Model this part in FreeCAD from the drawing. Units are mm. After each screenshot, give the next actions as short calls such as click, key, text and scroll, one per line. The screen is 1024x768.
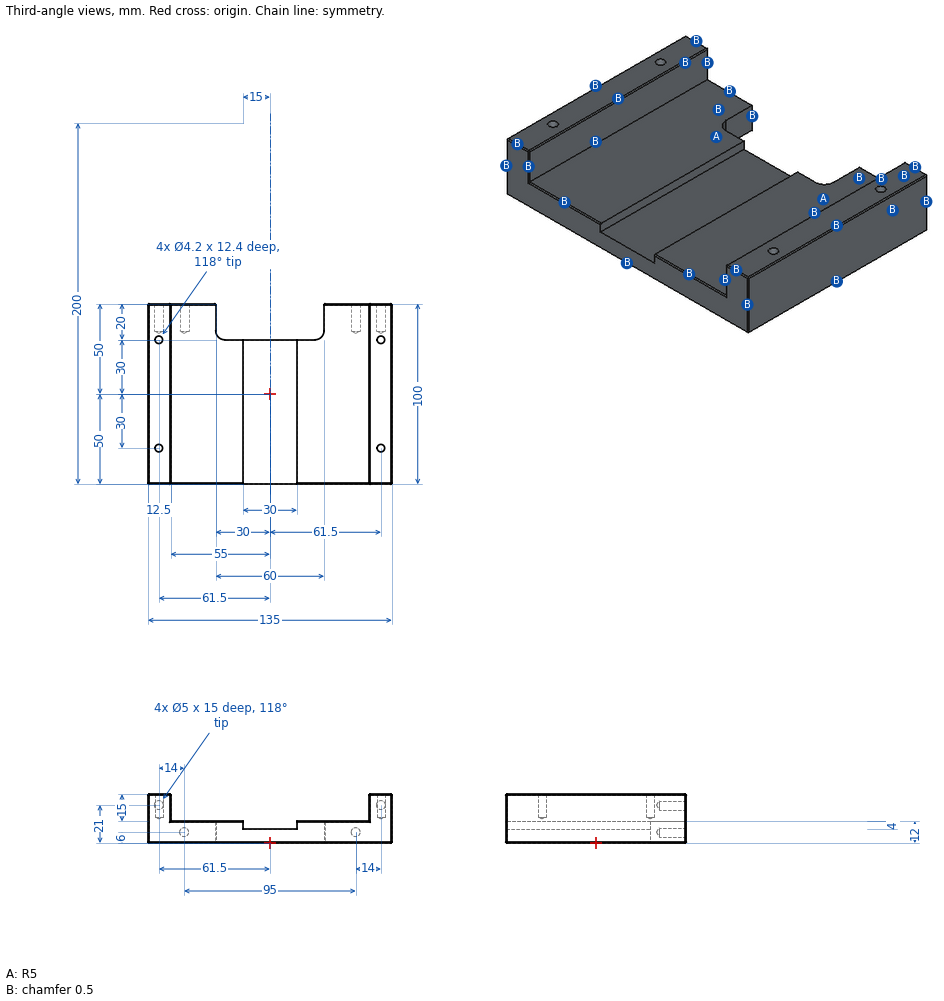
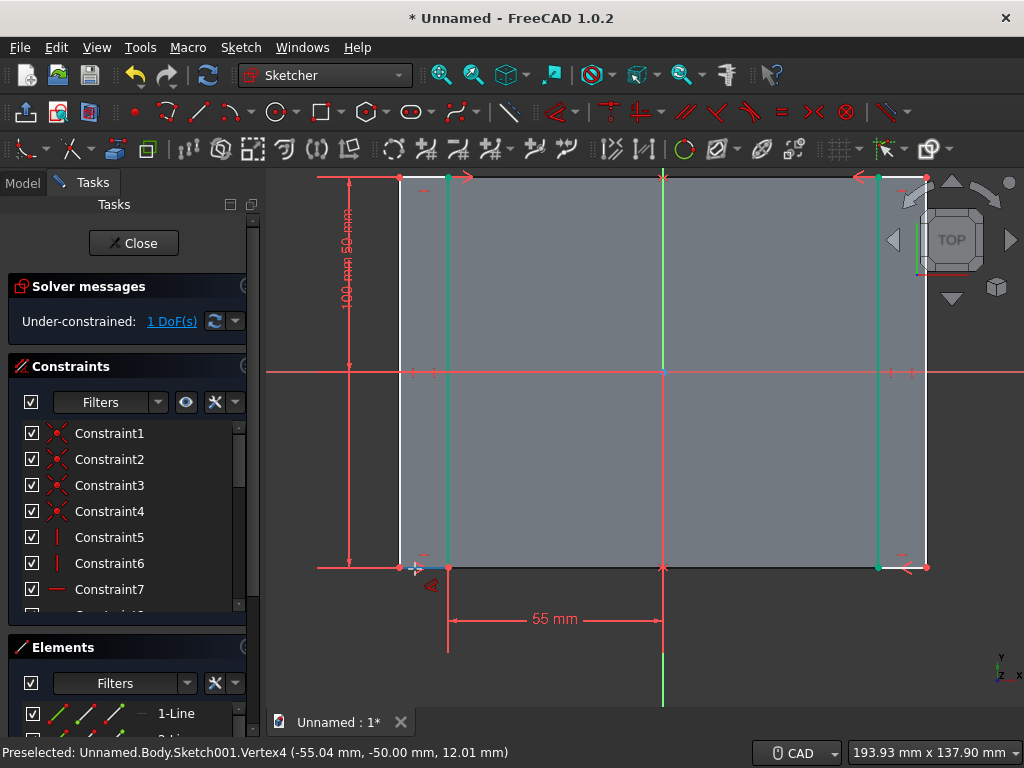
click(414, 568)
click(424, 602)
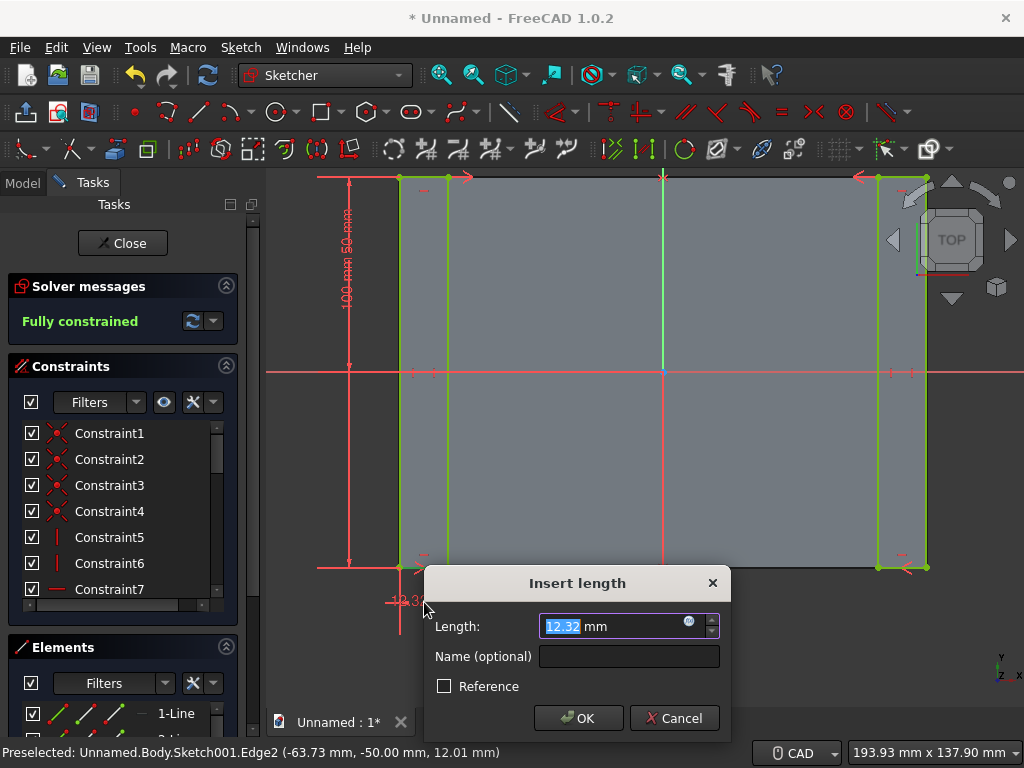
text(12.5)
key(Return)
key(Escape)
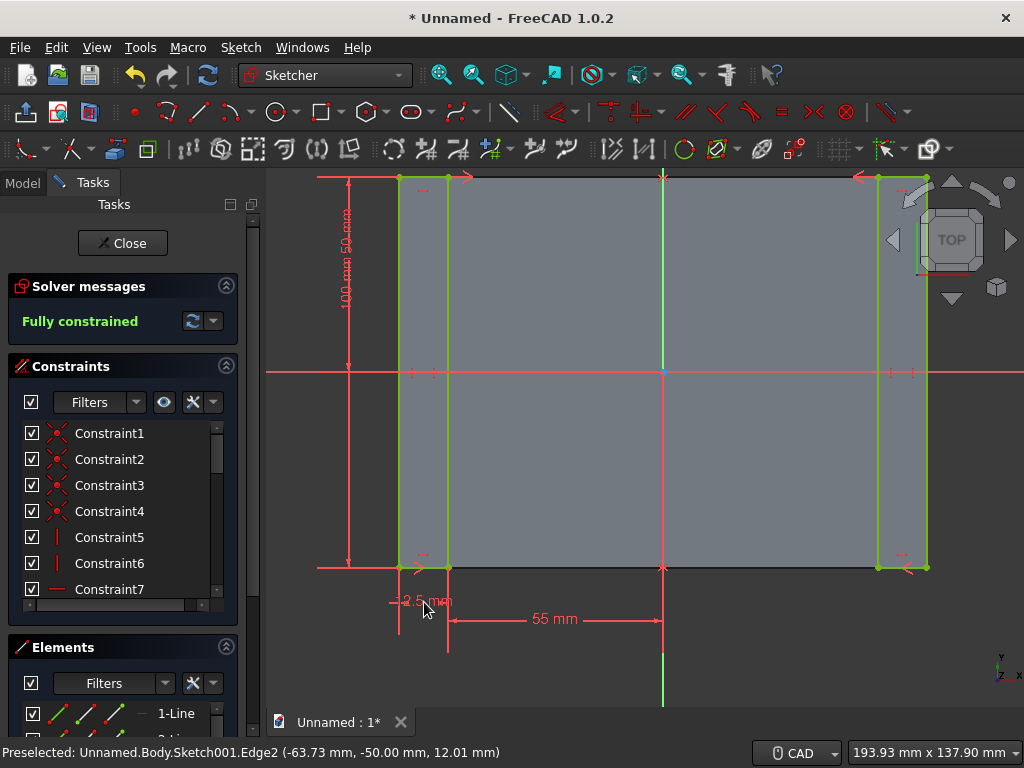
click(123, 243)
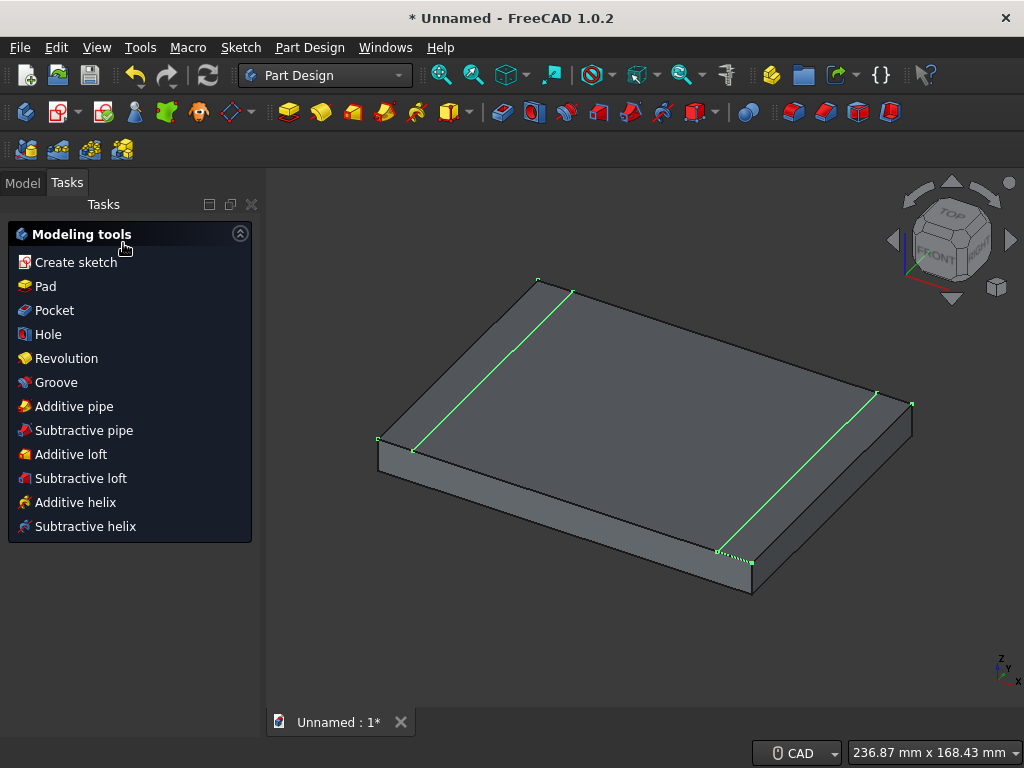
click(290, 112)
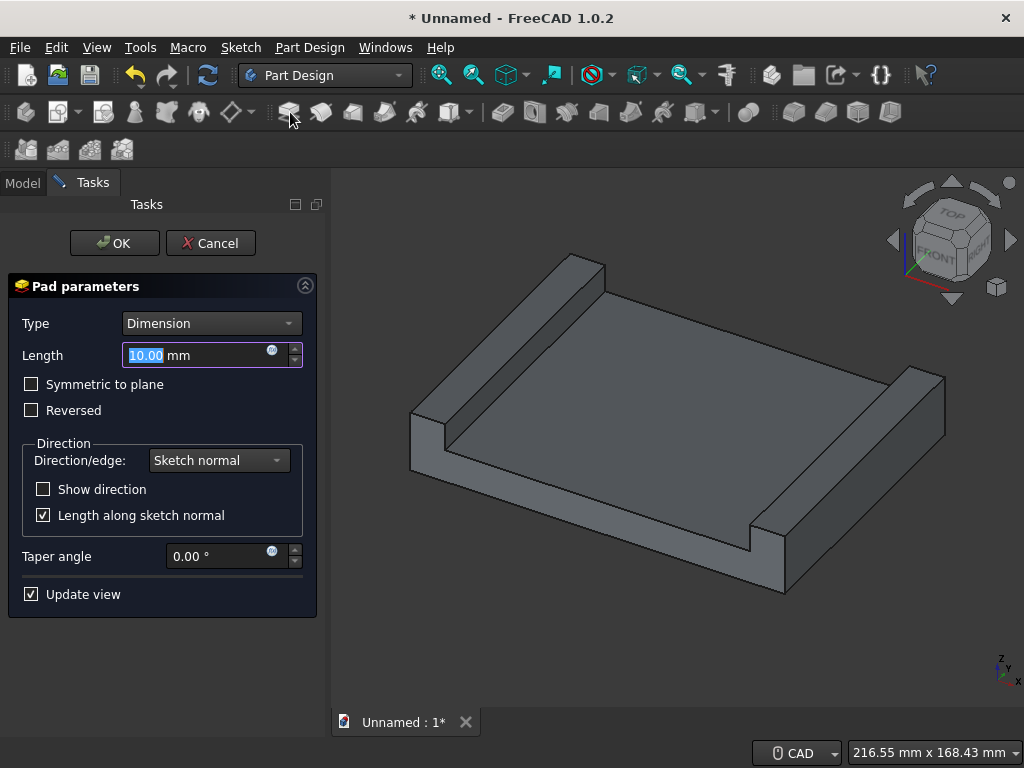
text(15)
key(Tab)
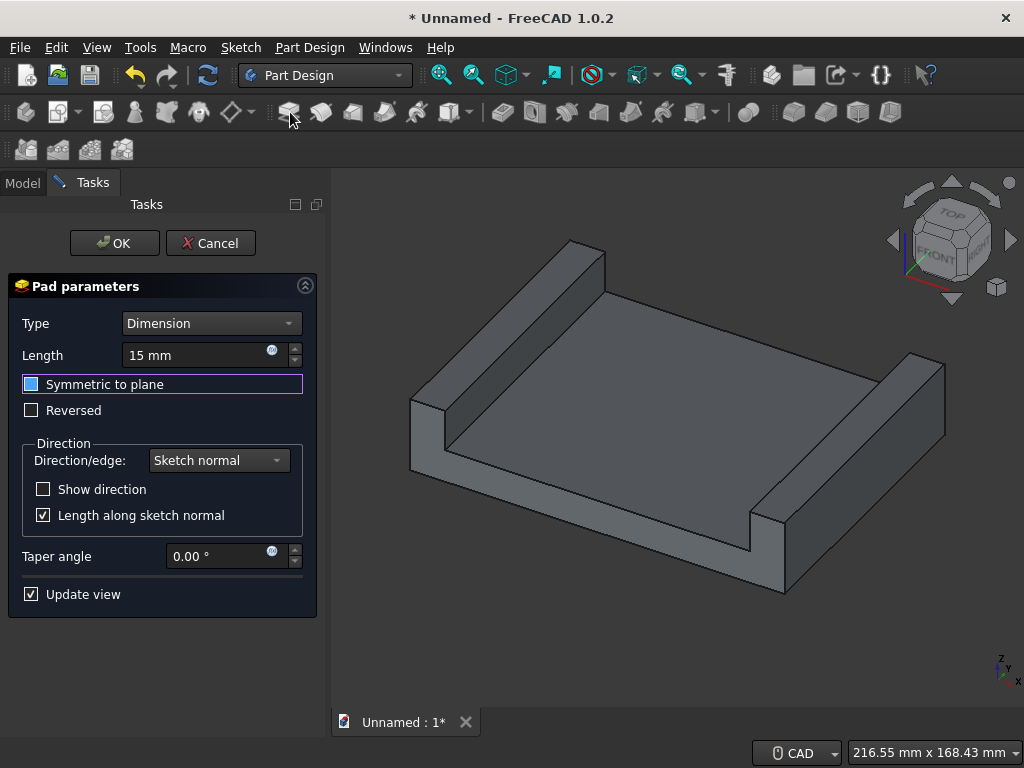
click(115, 243)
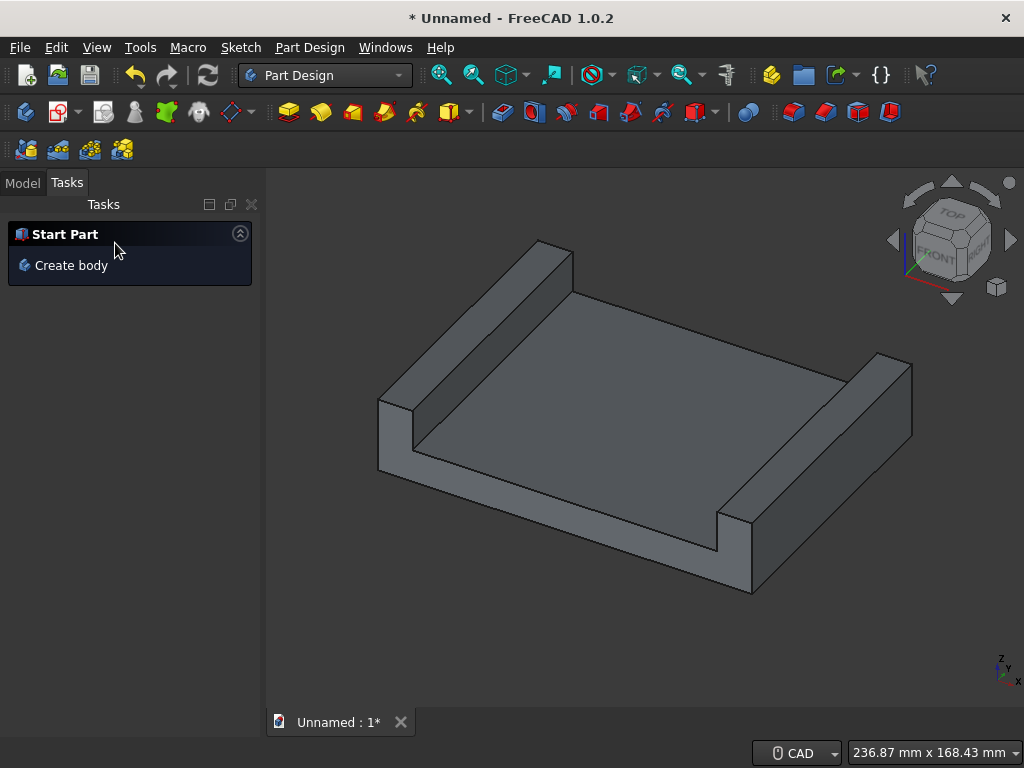
click(645, 420)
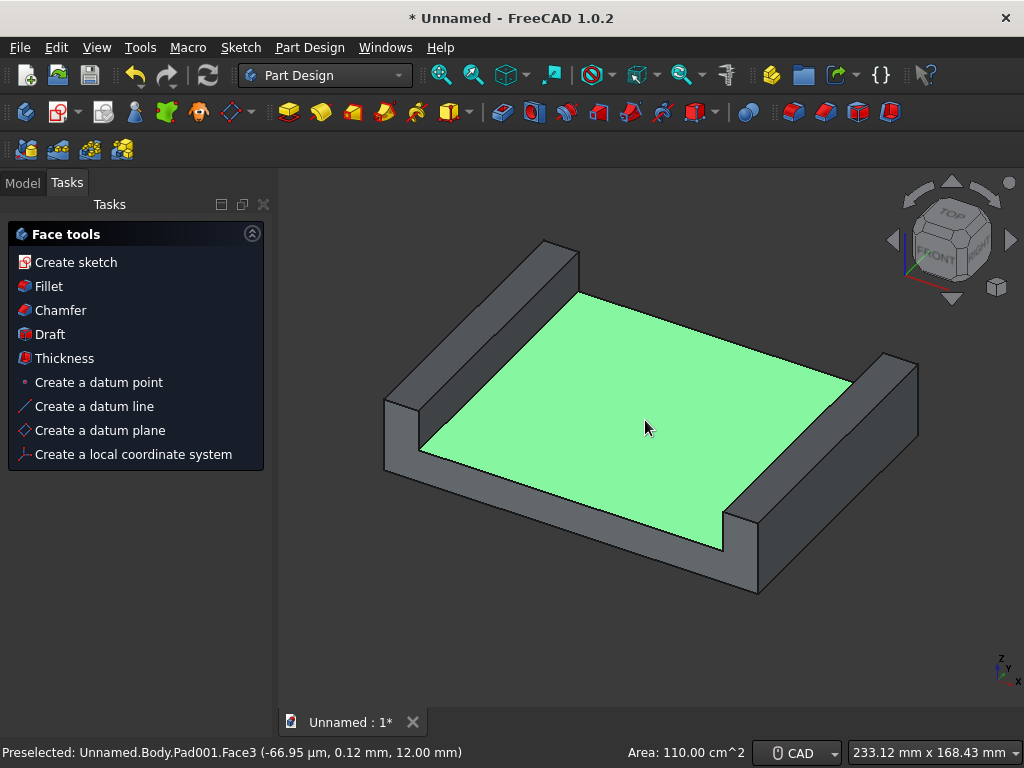
click(58, 112)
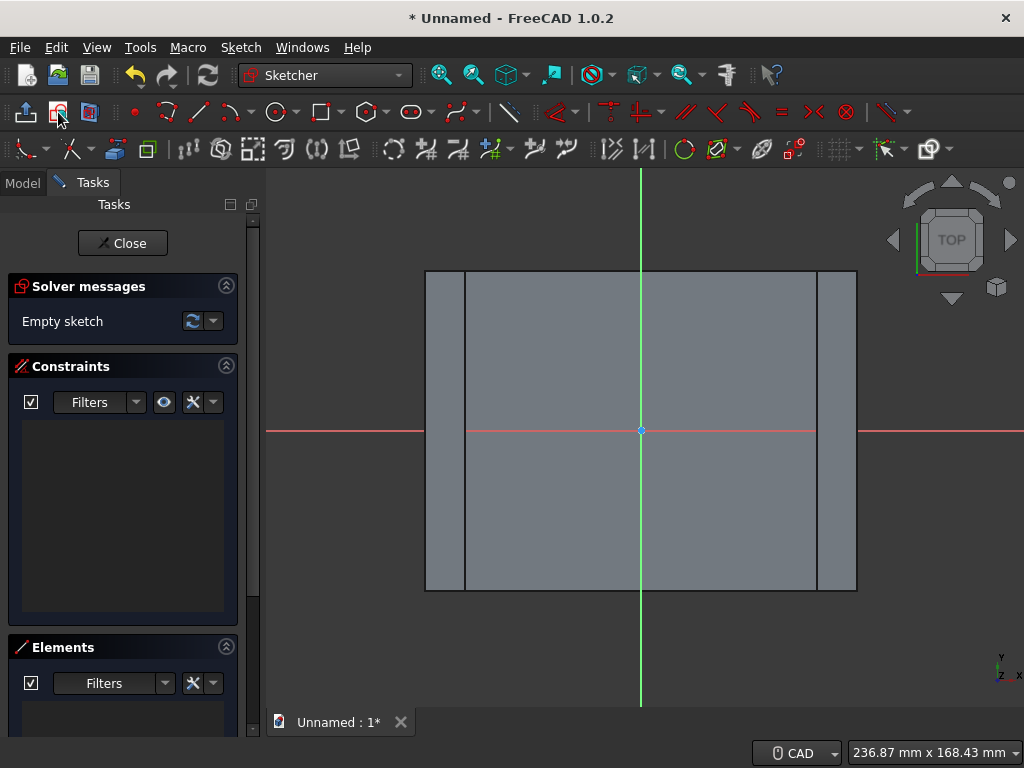
scroll(498, 640, down, 3)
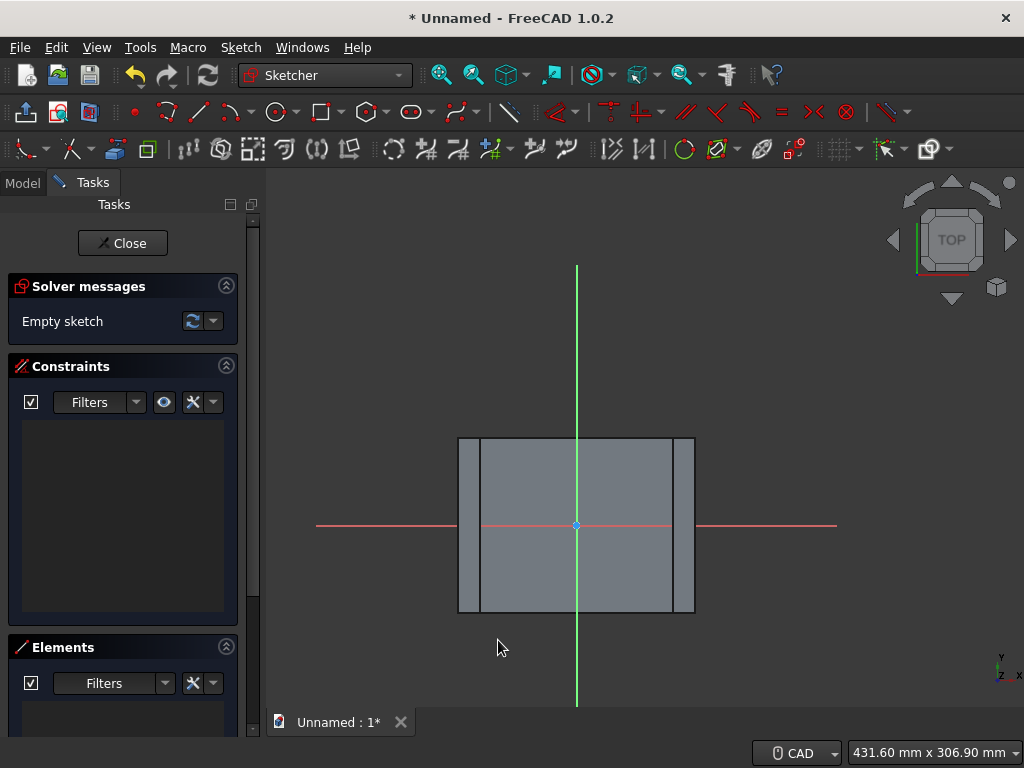
click(322, 112)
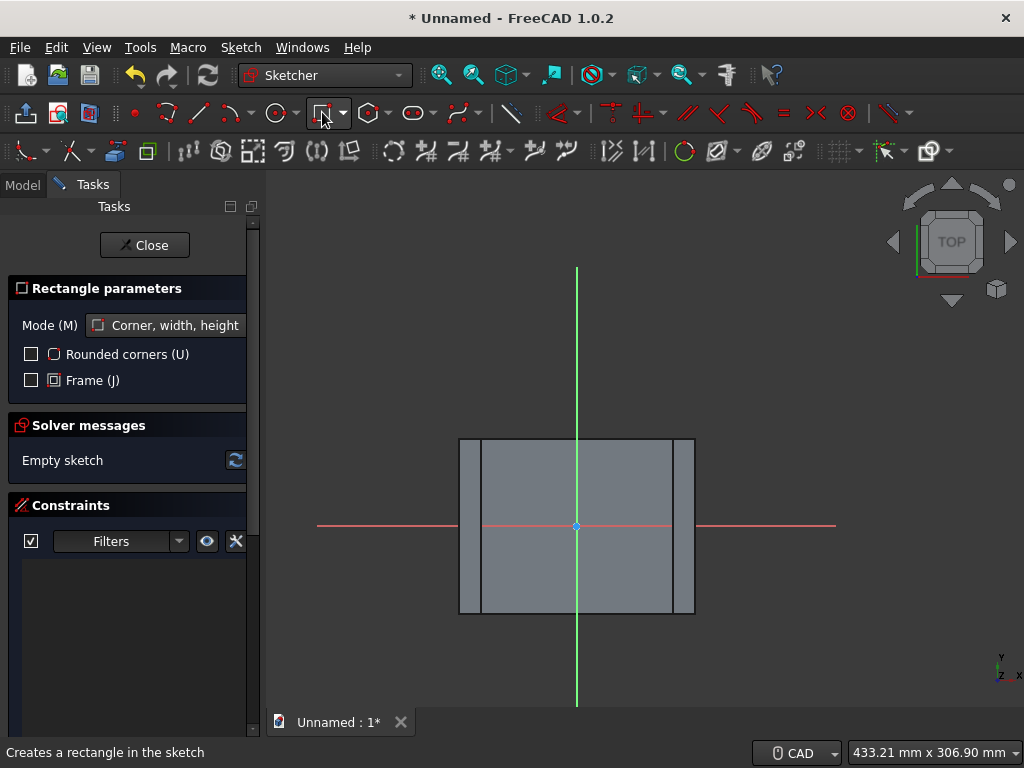
click(551, 264)
click(603, 614)
key(Escape)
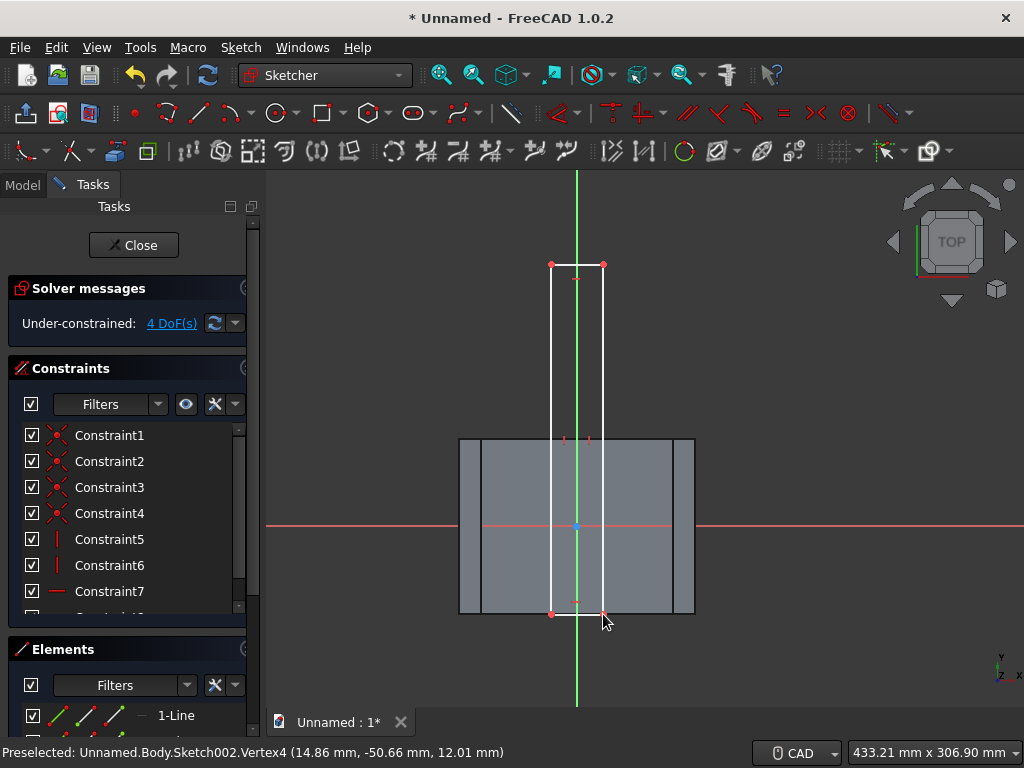
key(d)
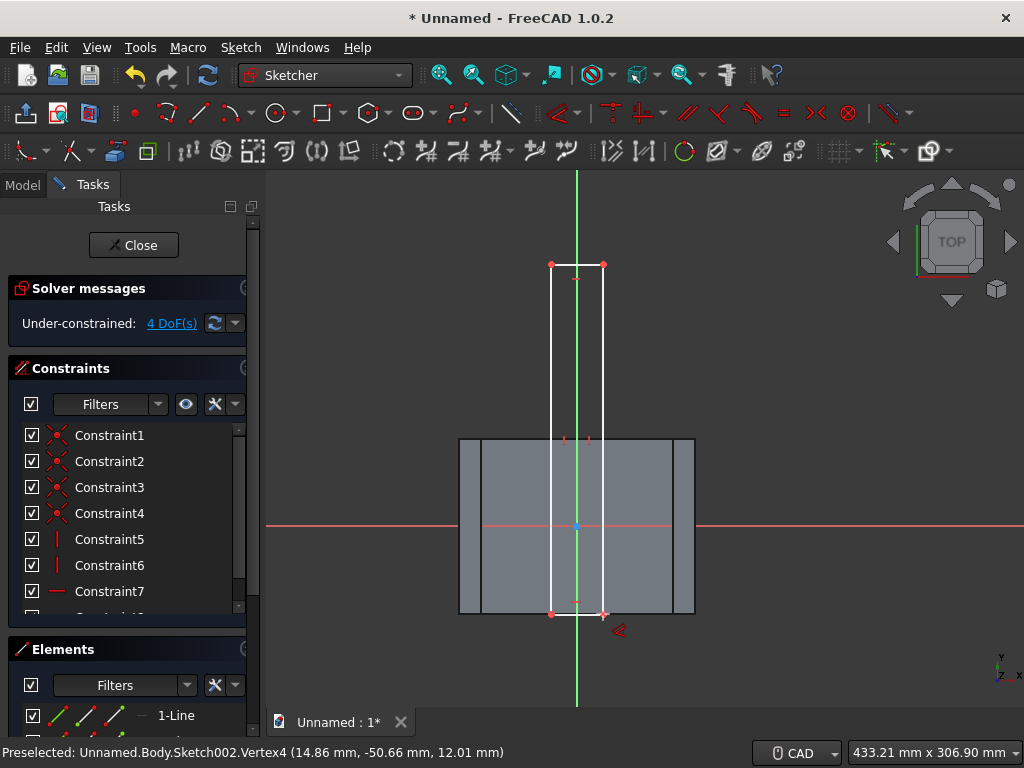
scroll(567, 615, up, 2)